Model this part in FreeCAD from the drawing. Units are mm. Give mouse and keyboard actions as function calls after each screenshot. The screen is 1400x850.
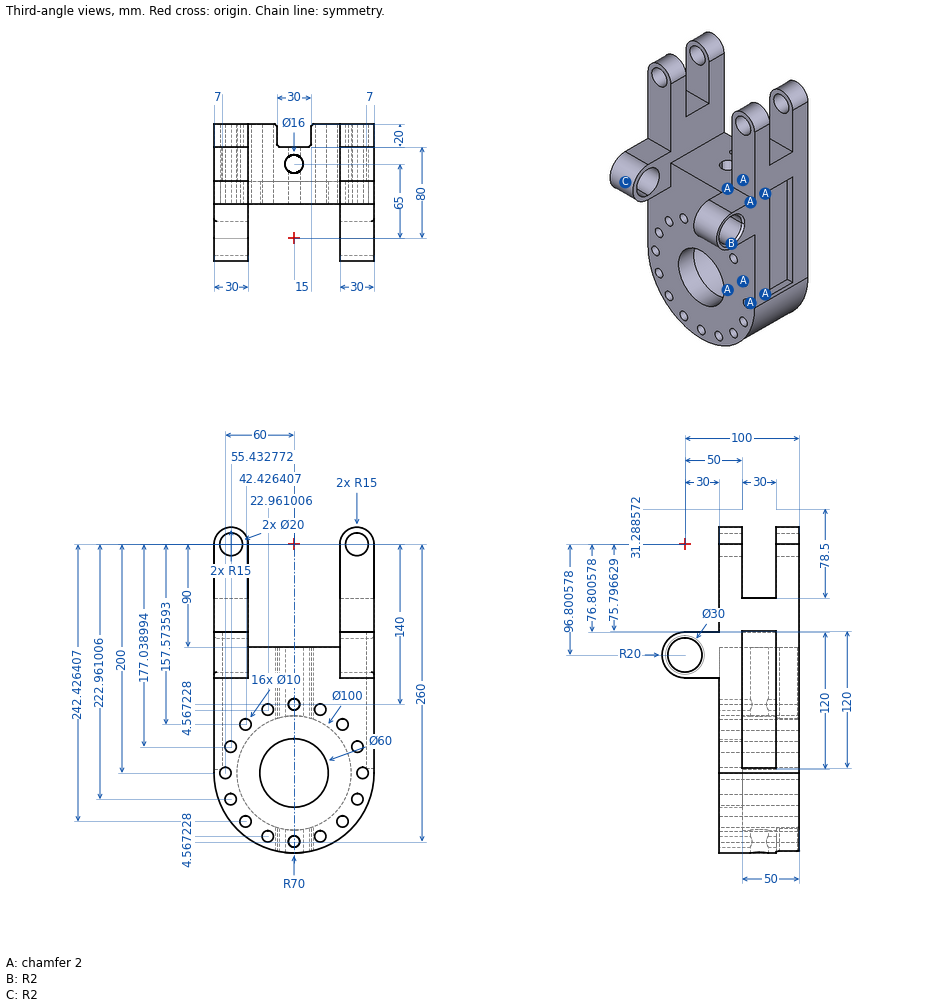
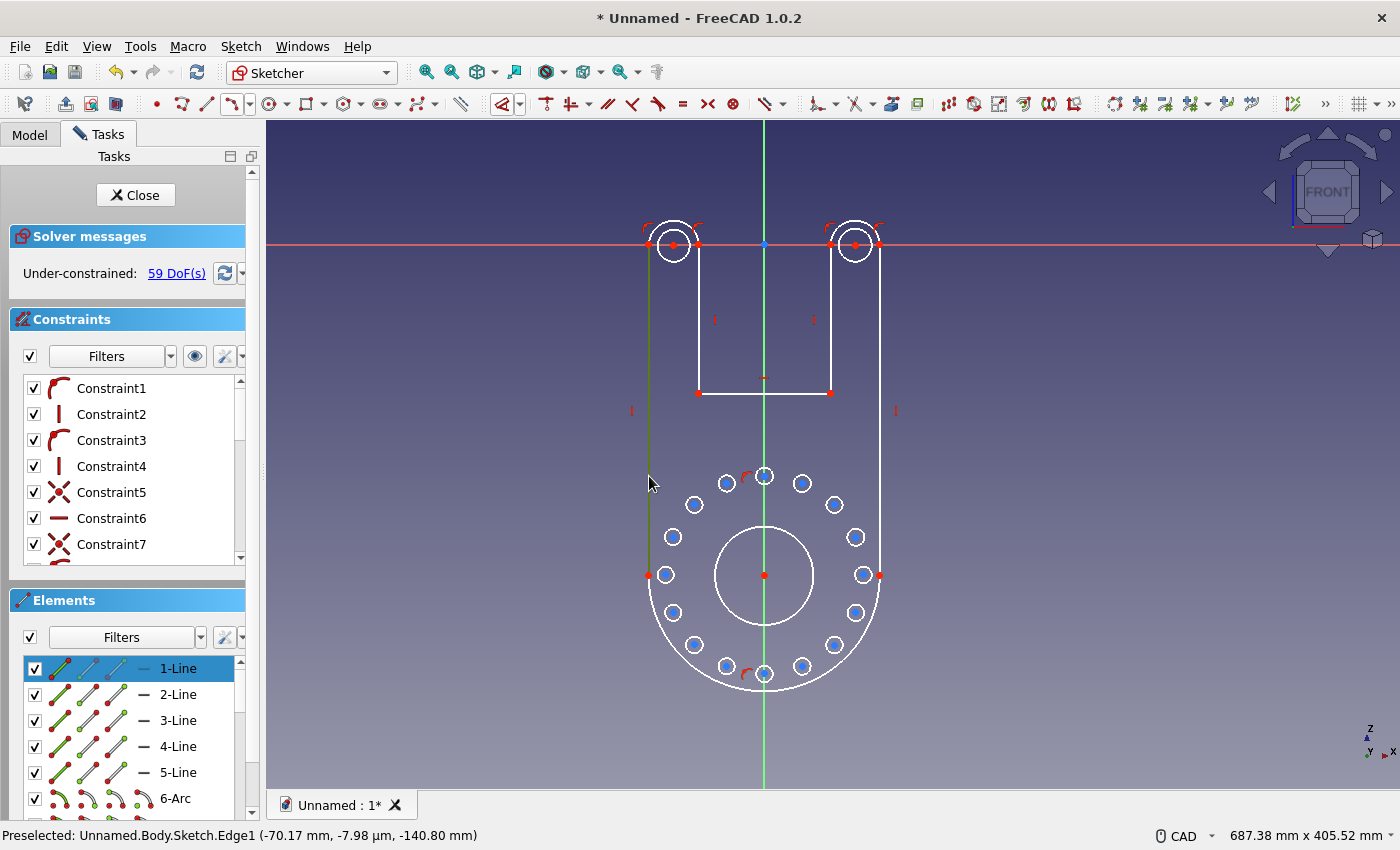
scroll(688, 225, up, 3)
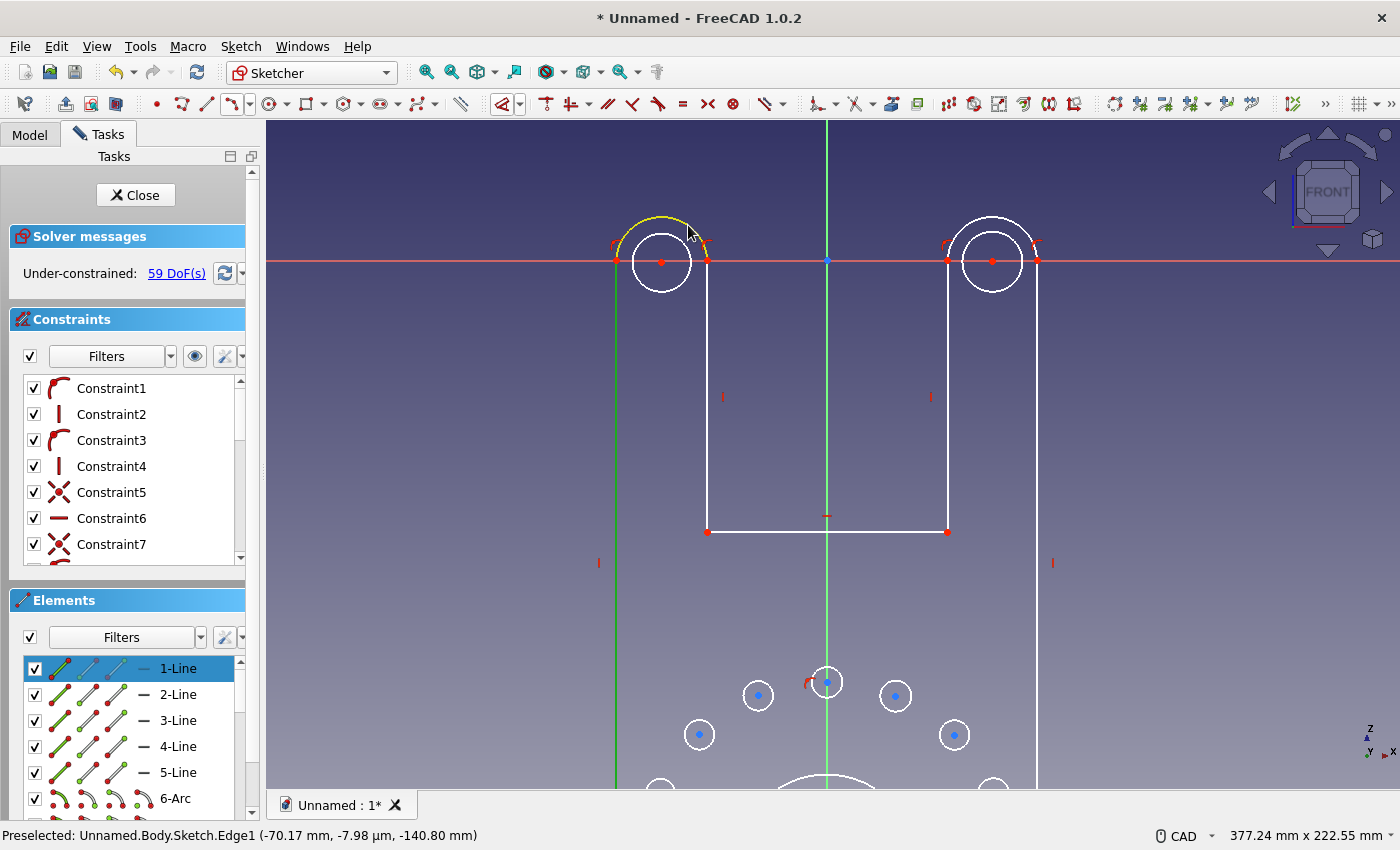
click(688, 225)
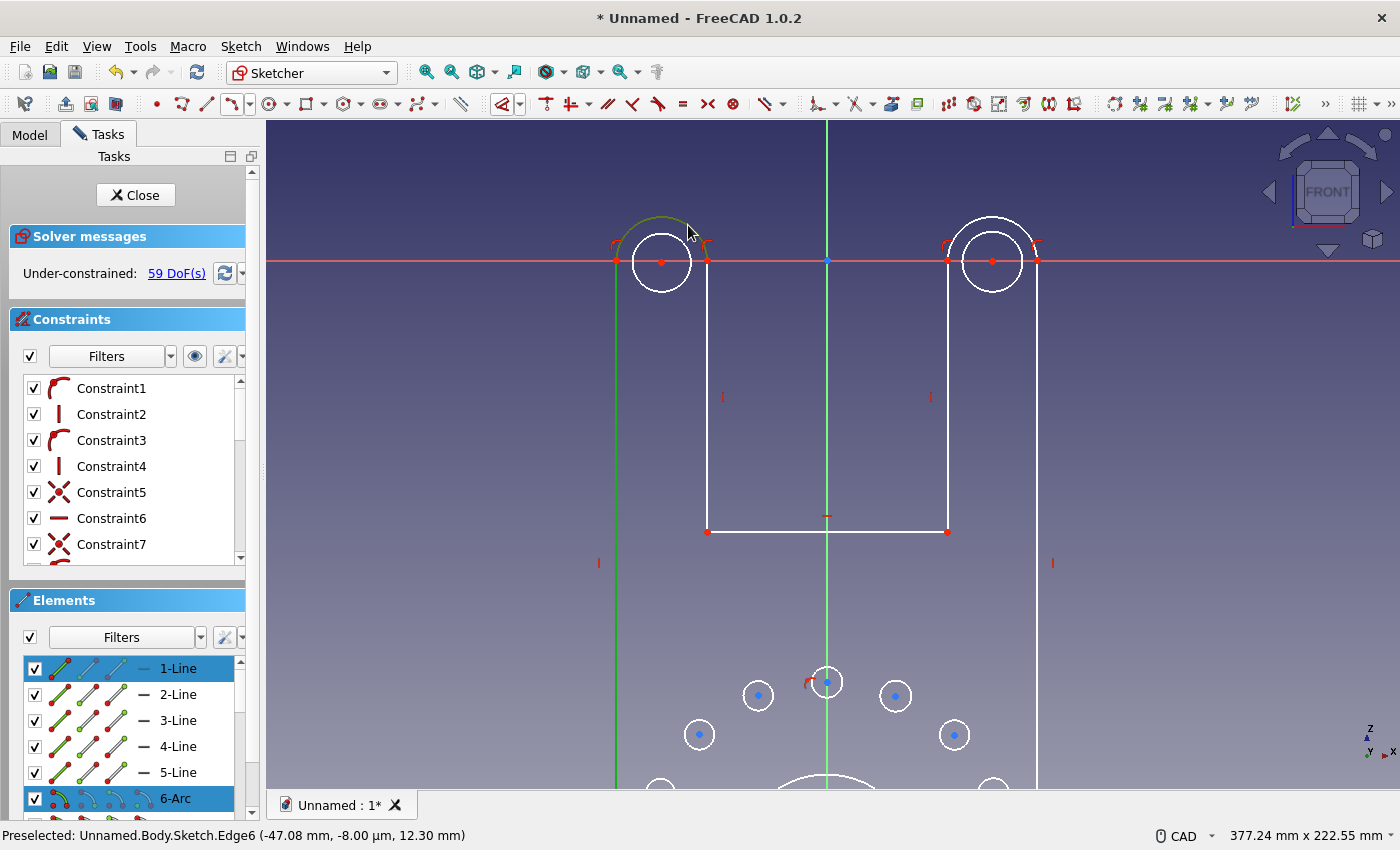
key(t)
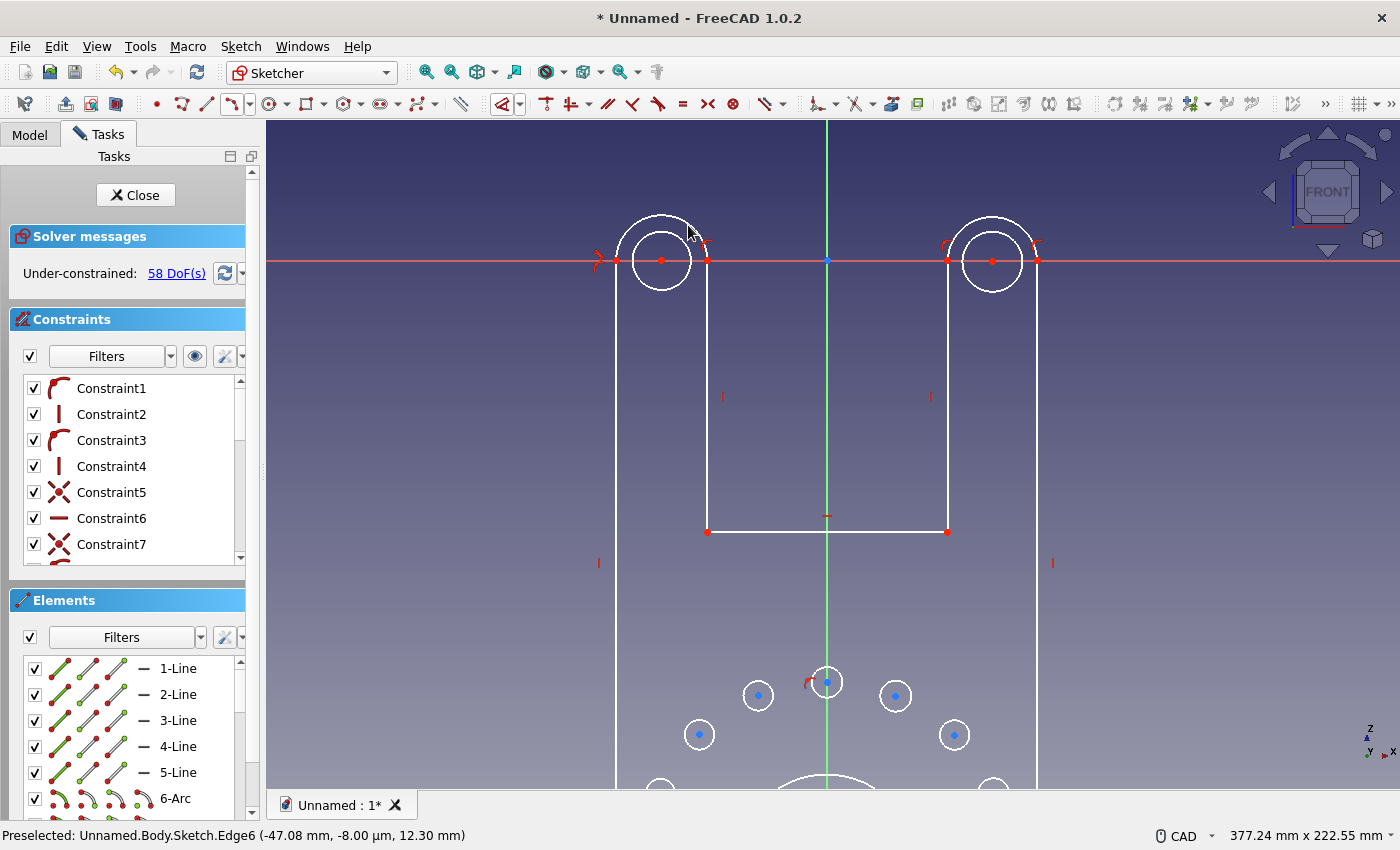
click(948, 451)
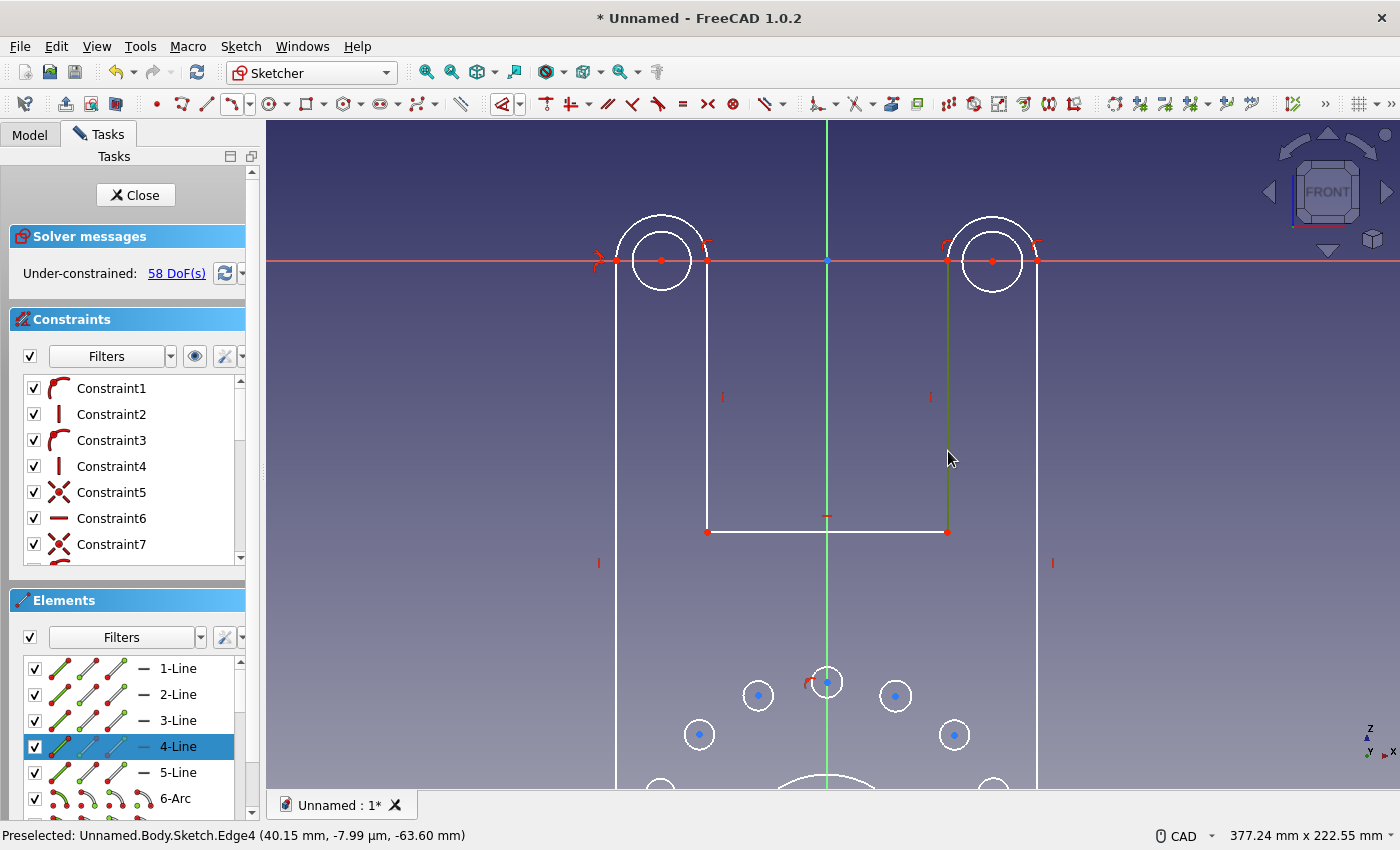
click(1018, 225)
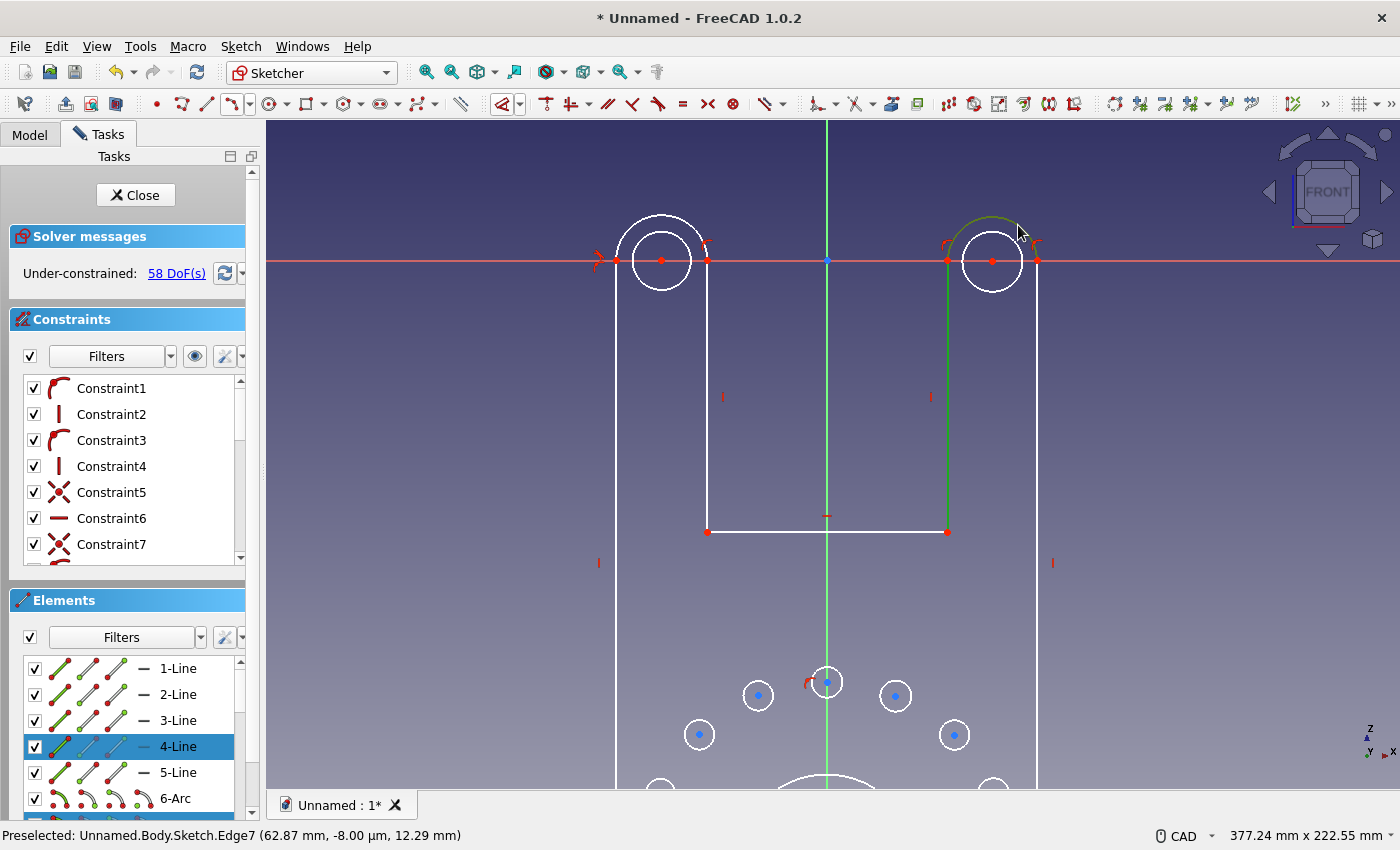
key(t)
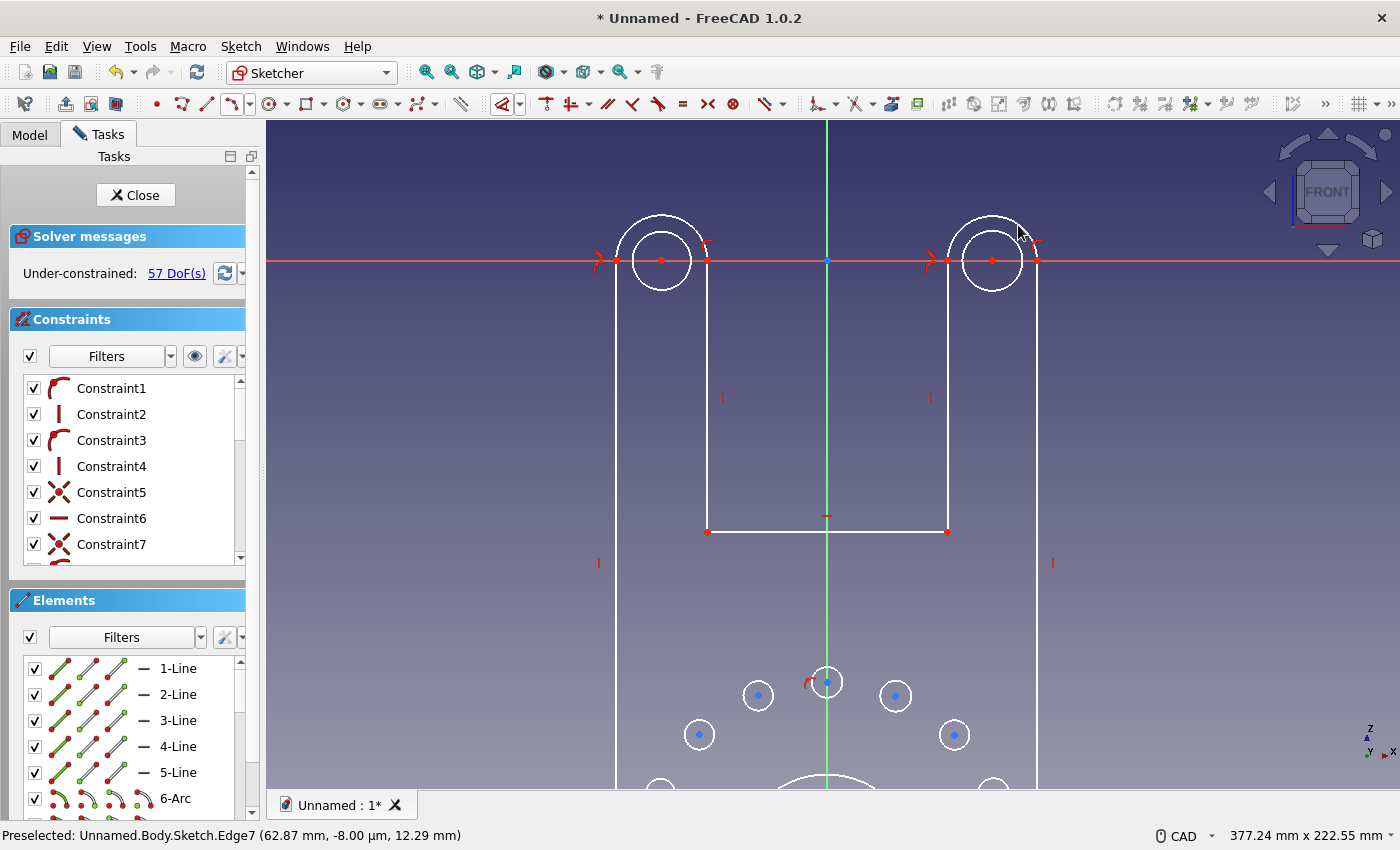
click(688, 224)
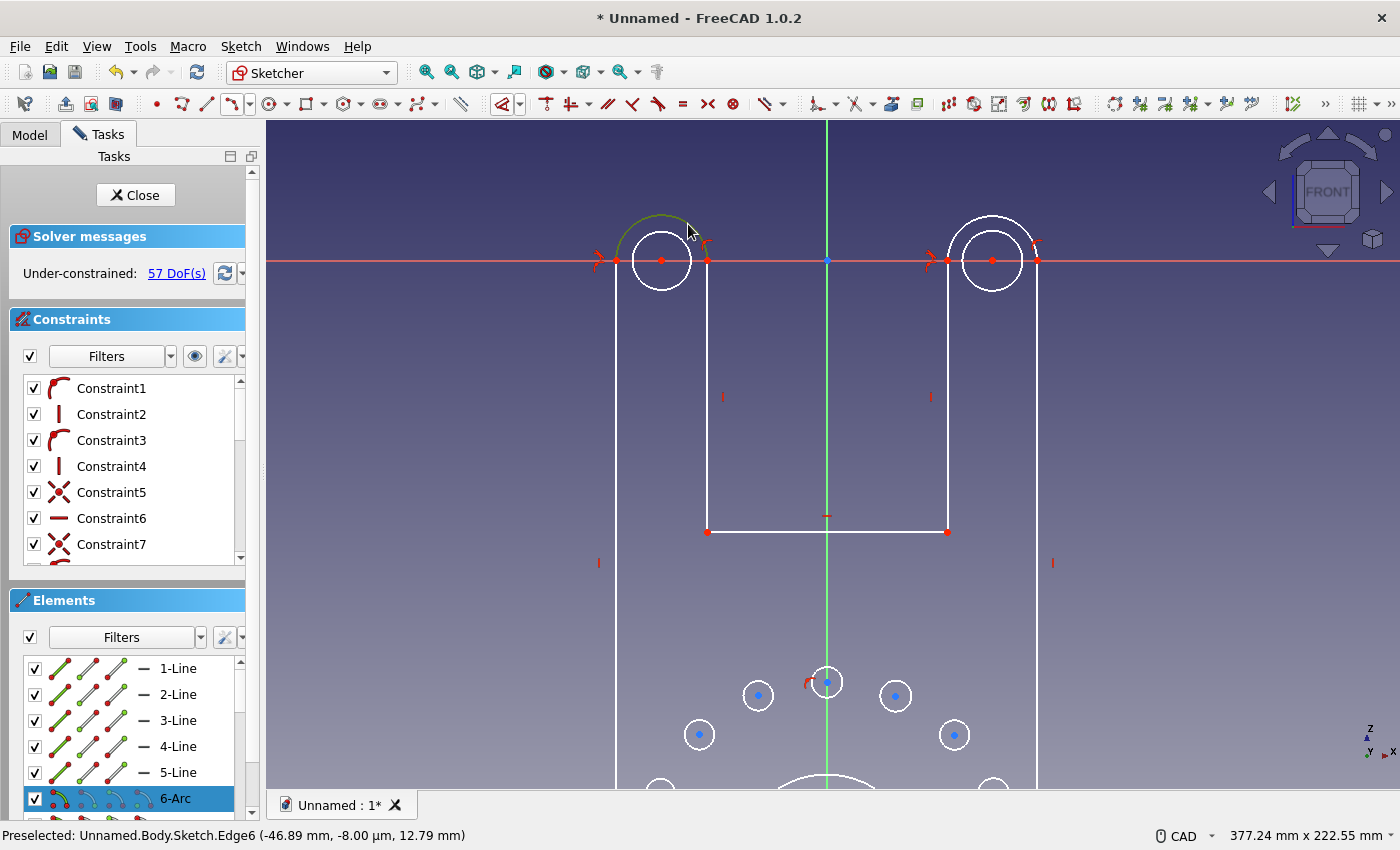
click(1019, 225)